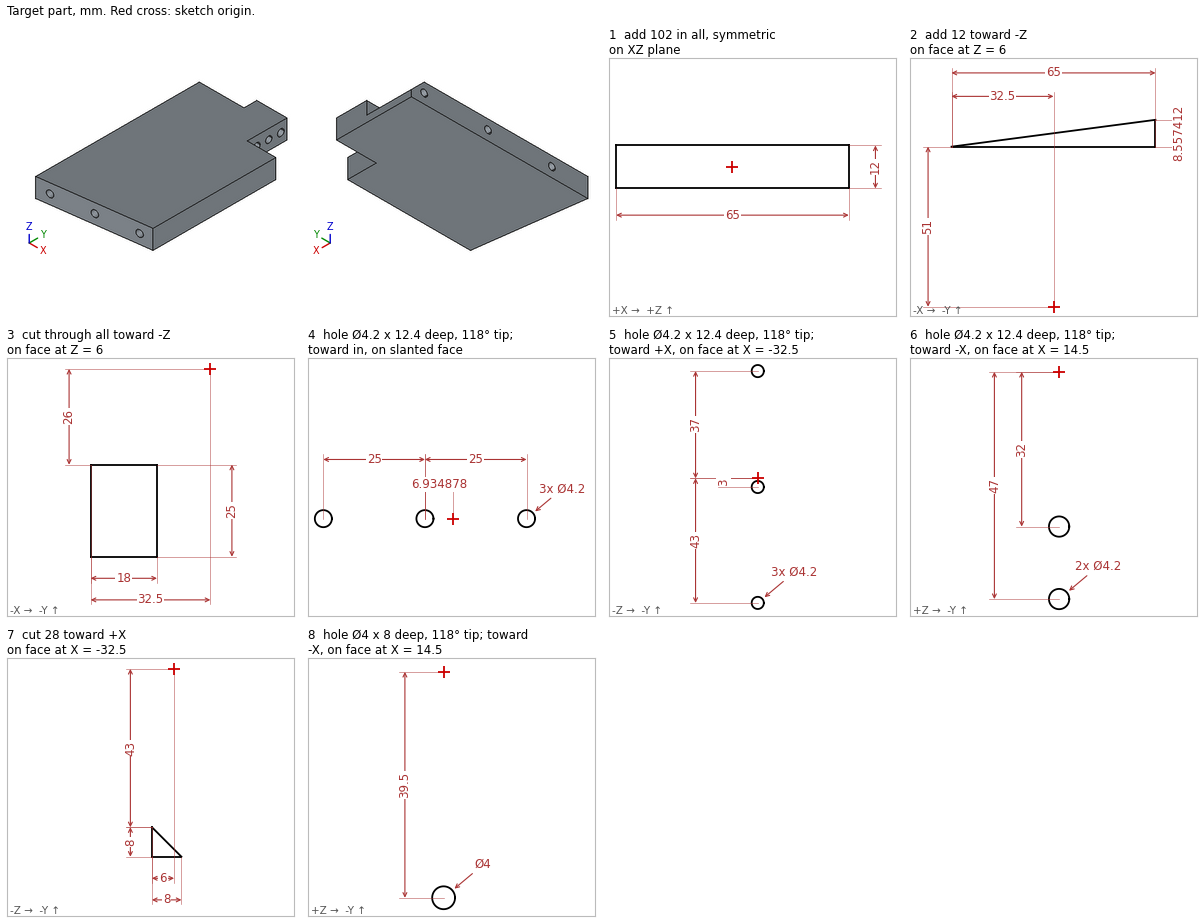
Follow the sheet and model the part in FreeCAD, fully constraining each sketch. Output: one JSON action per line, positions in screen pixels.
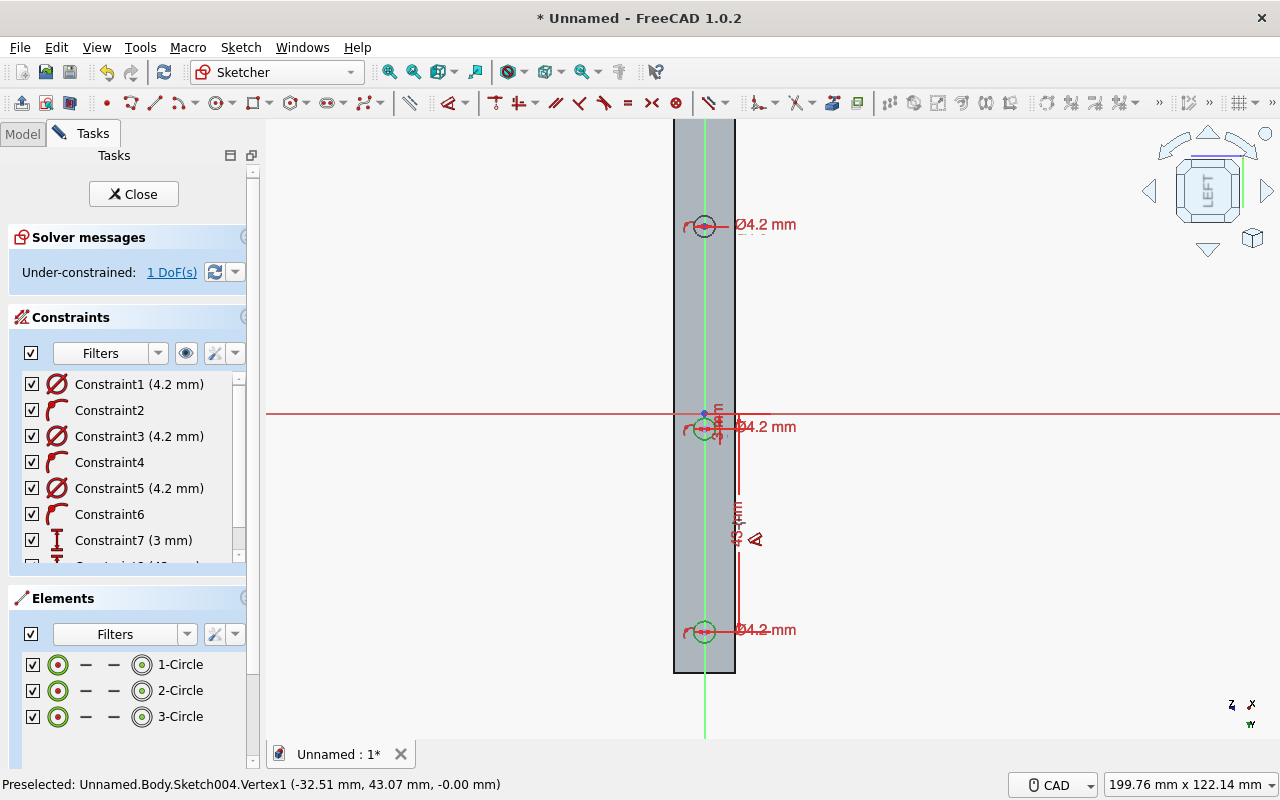
{"action": "left_click", "coordinate": [705, 227]}
{"action": "left_click", "coordinate": [739, 320]}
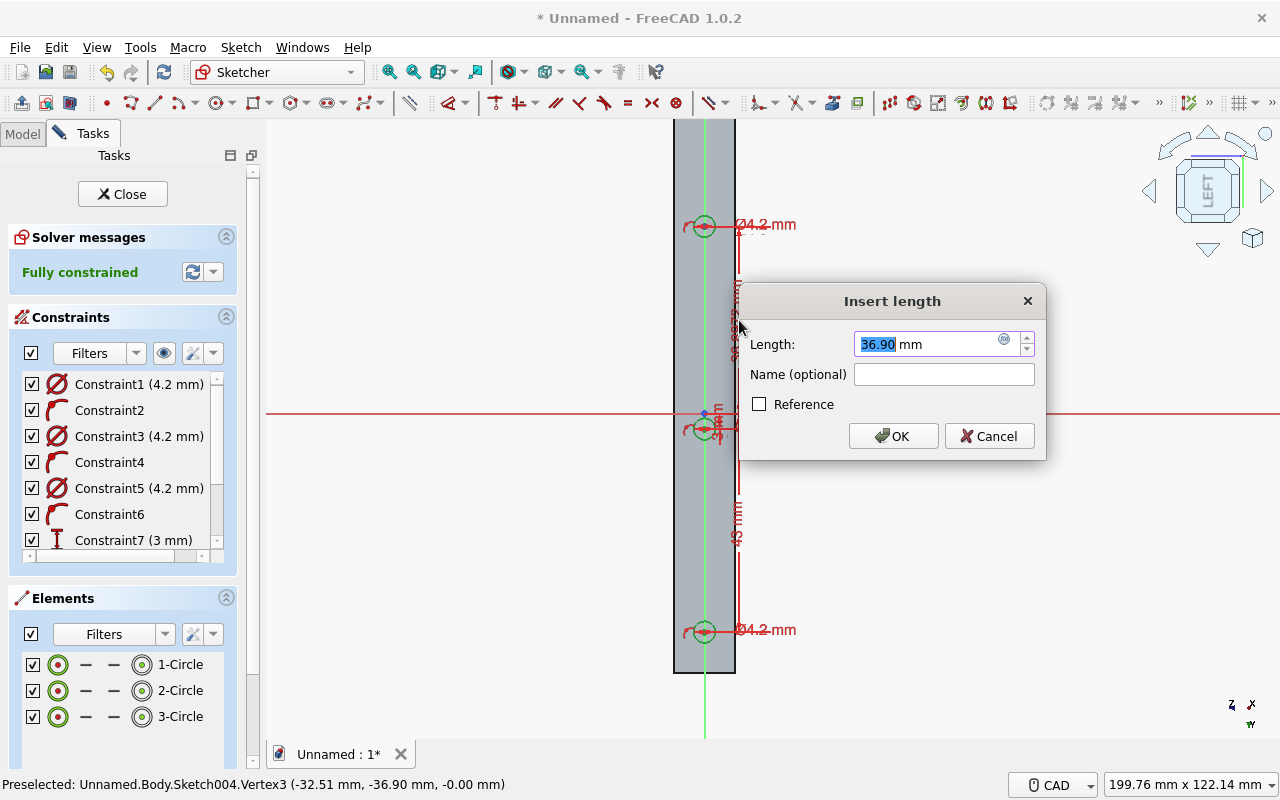
{"action": "type", "text": "37"}
{"action": "key", "text": "Return"}
{"action": "key", "text": "Escape"}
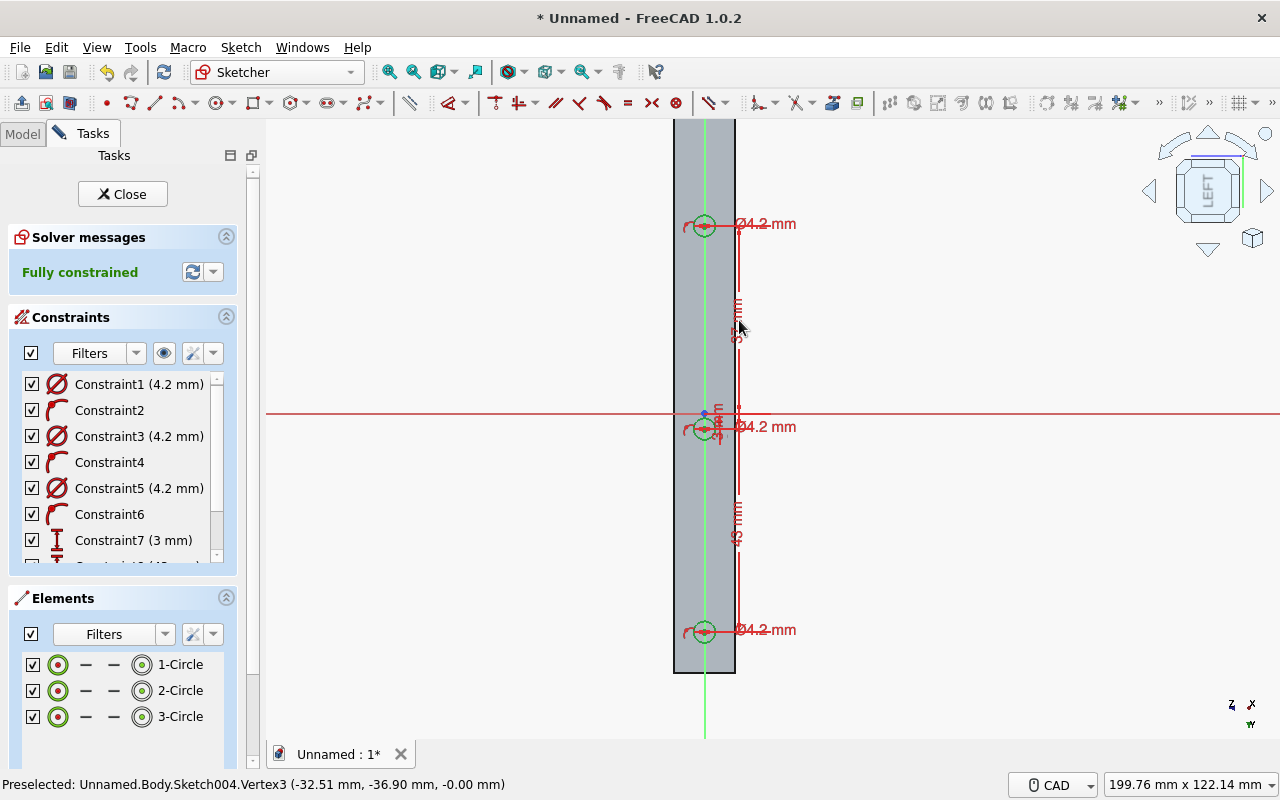
{"action": "left_click", "coordinate": [123, 194]}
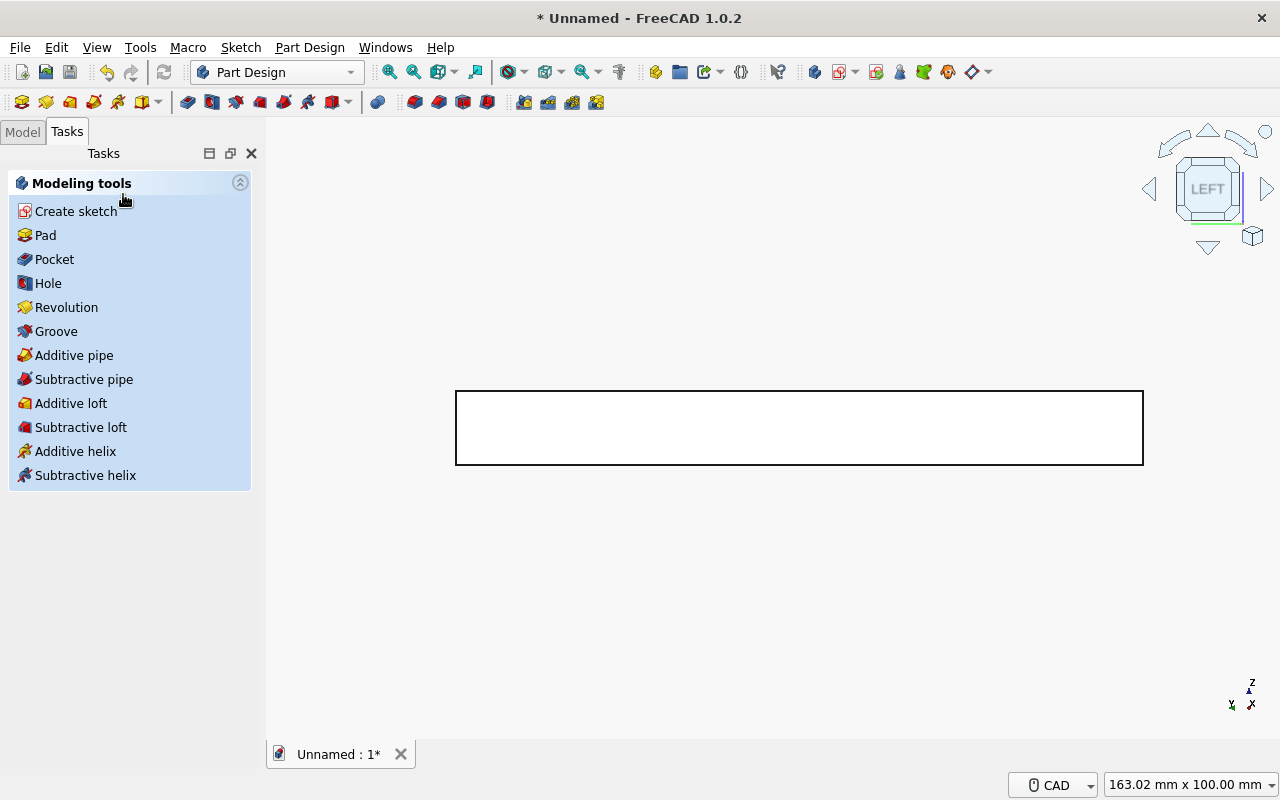
{"action": "left_click", "coordinate": [212, 102]}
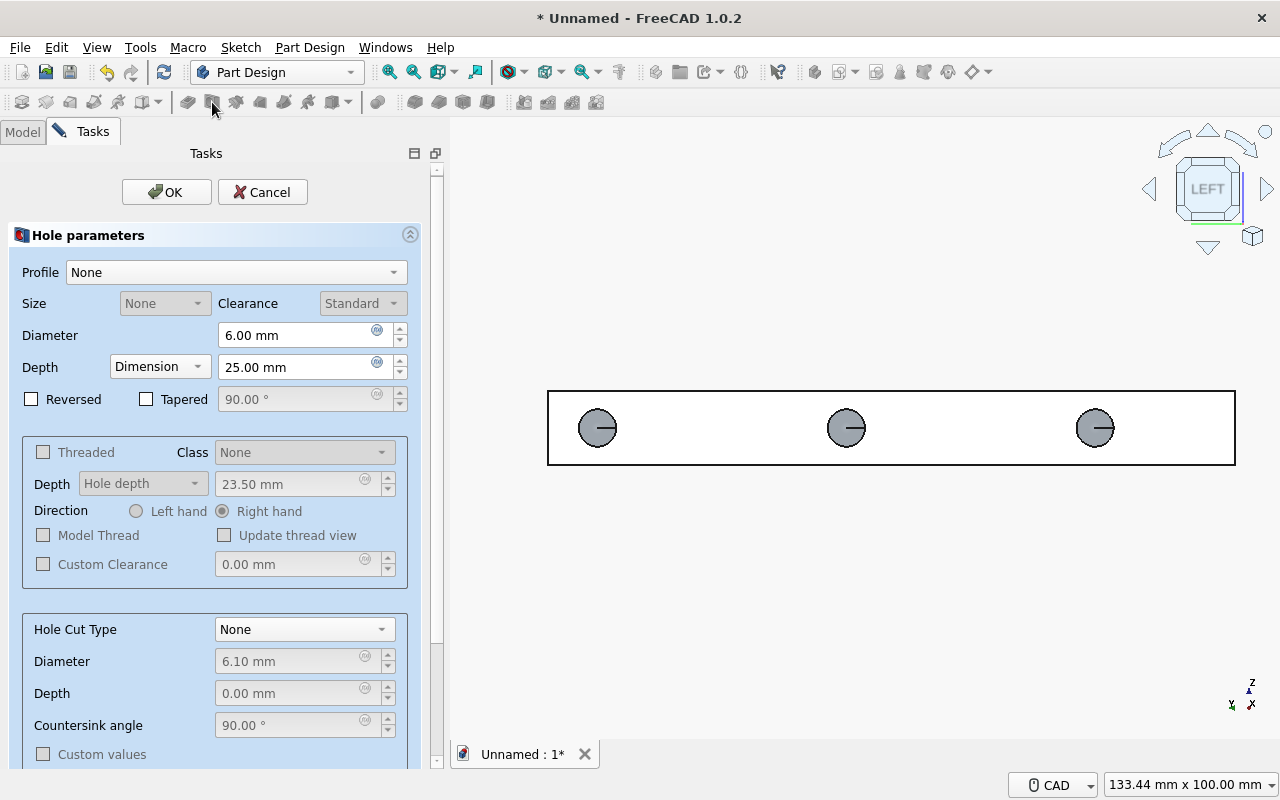
{"action": "triple_click", "coordinate": [305, 335]}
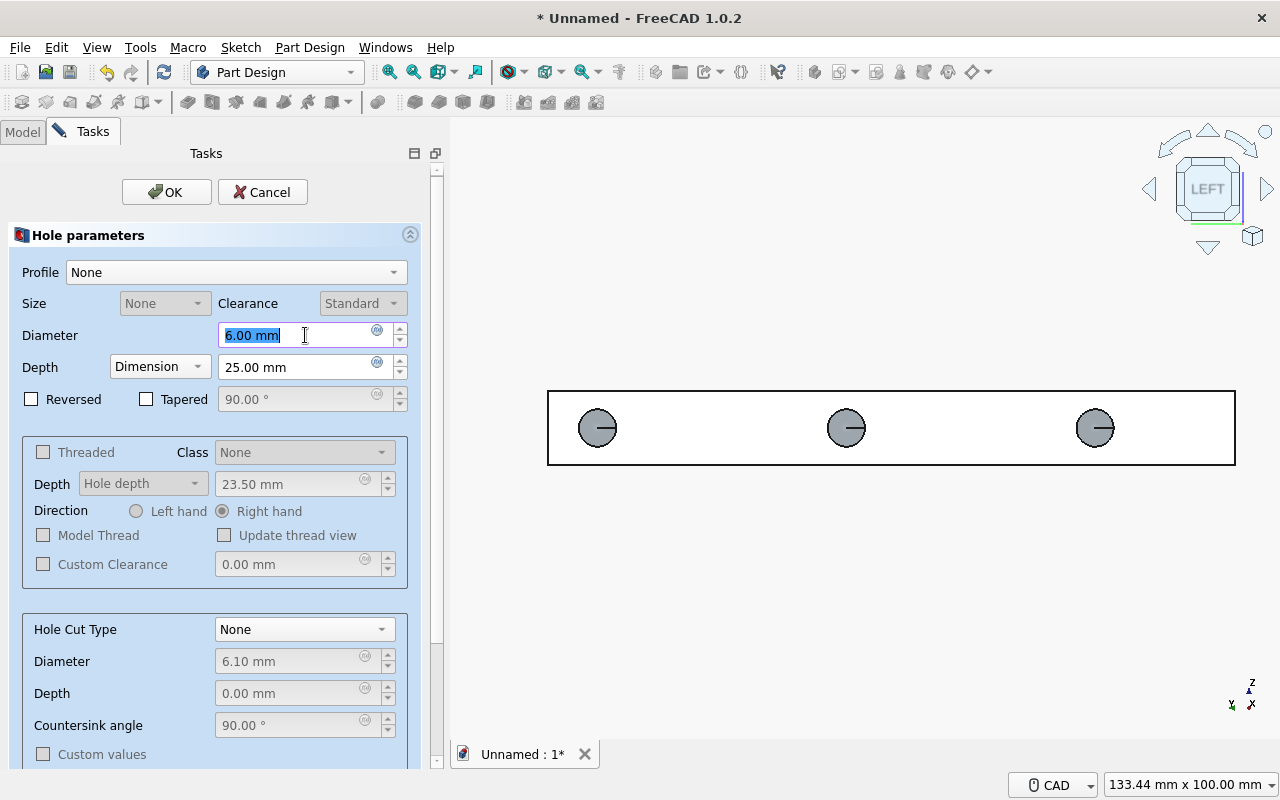
{"action": "type", "text": "4.2"}
{"action": "key", "text": "Tab"}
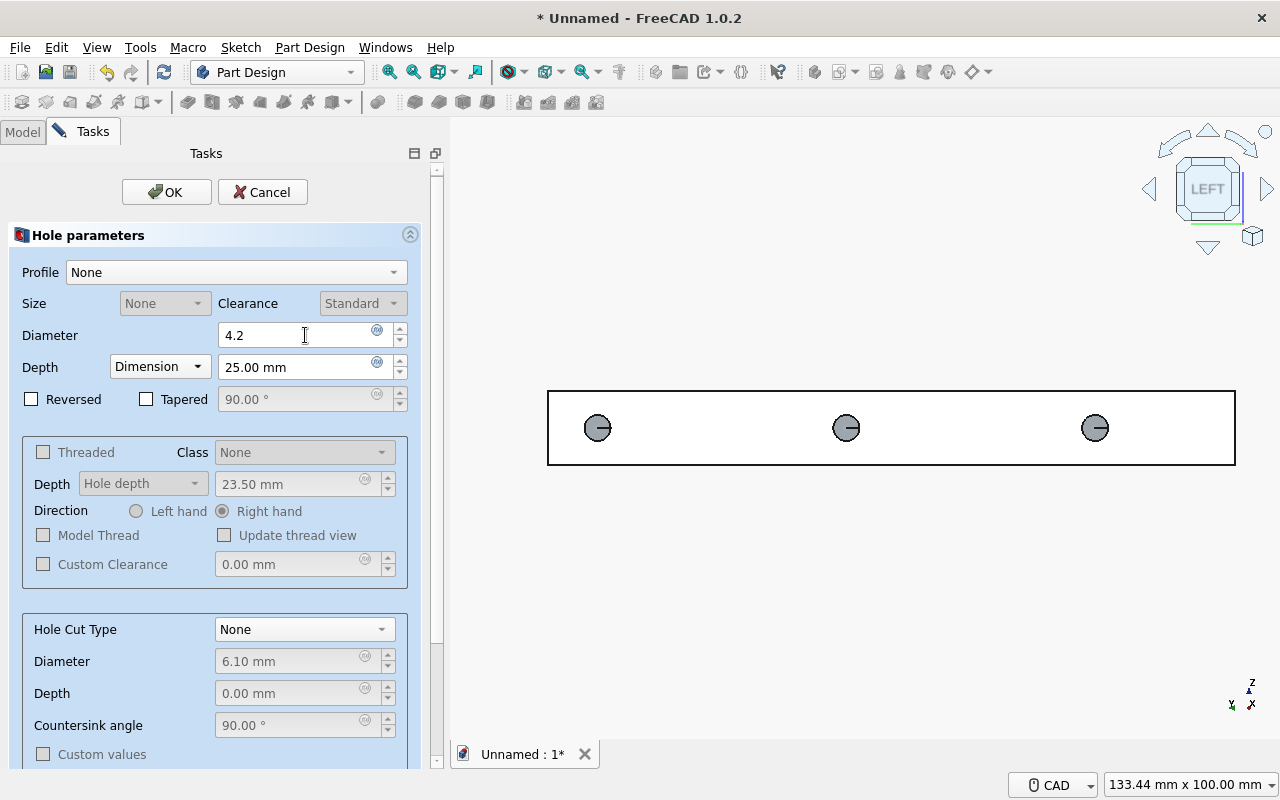
{"action": "triple_click", "coordinate": [305, 367]}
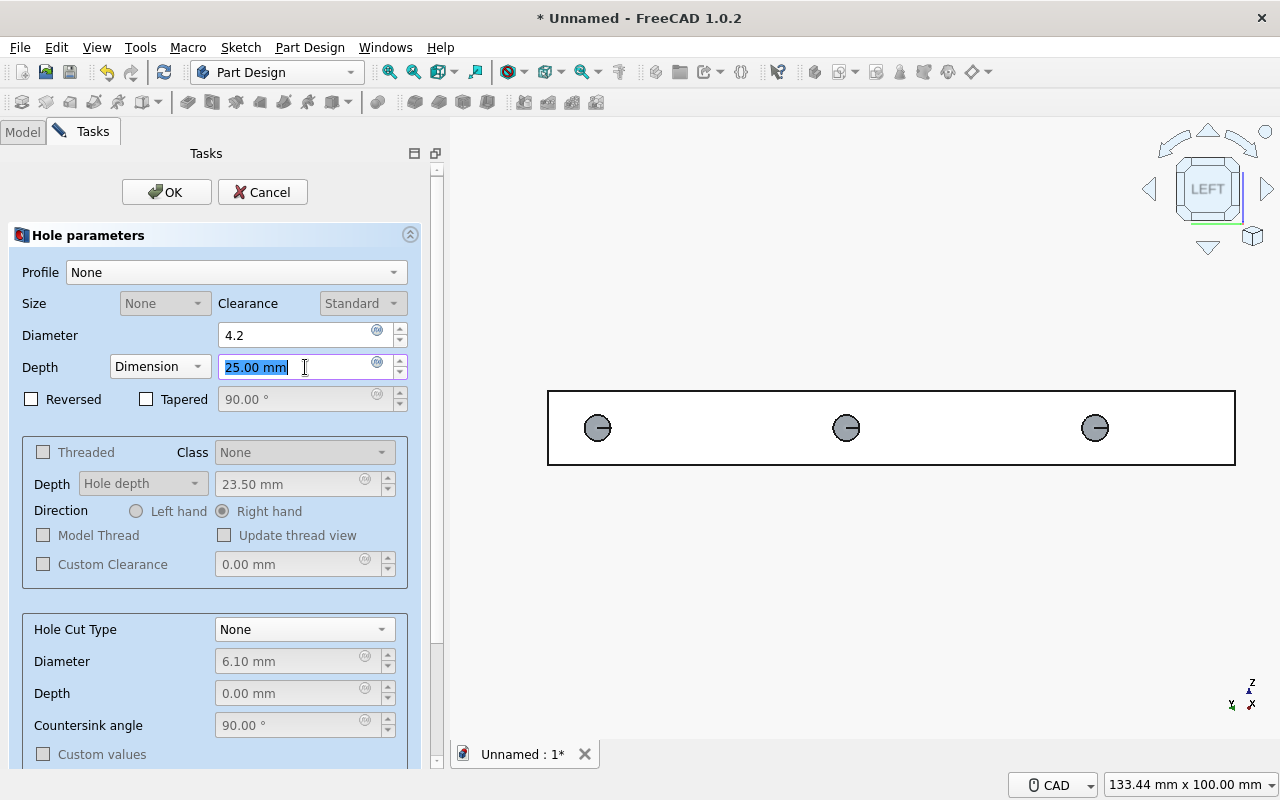
{"action": "type", "text": "12.4"}
{"action": "key", "text": "Tab"}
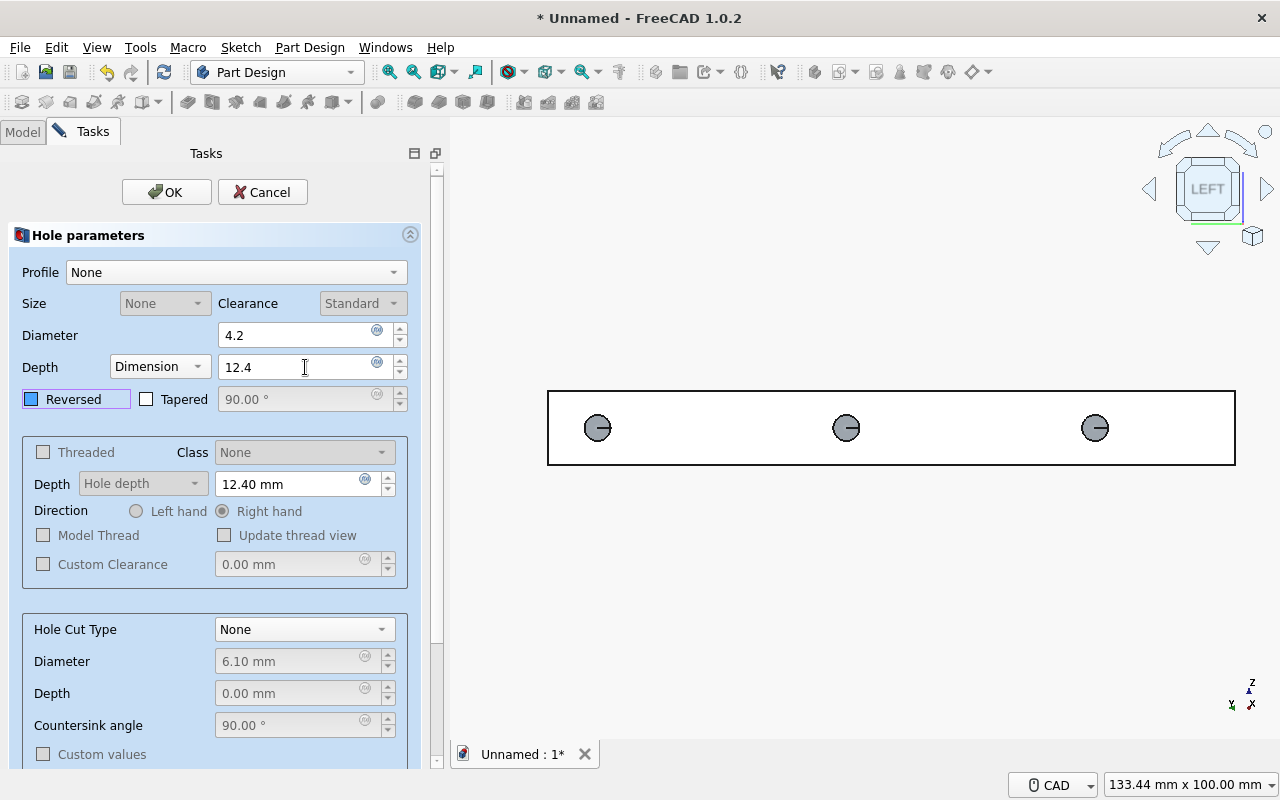
{"action": "left_click", "coordinate": [167, 192]}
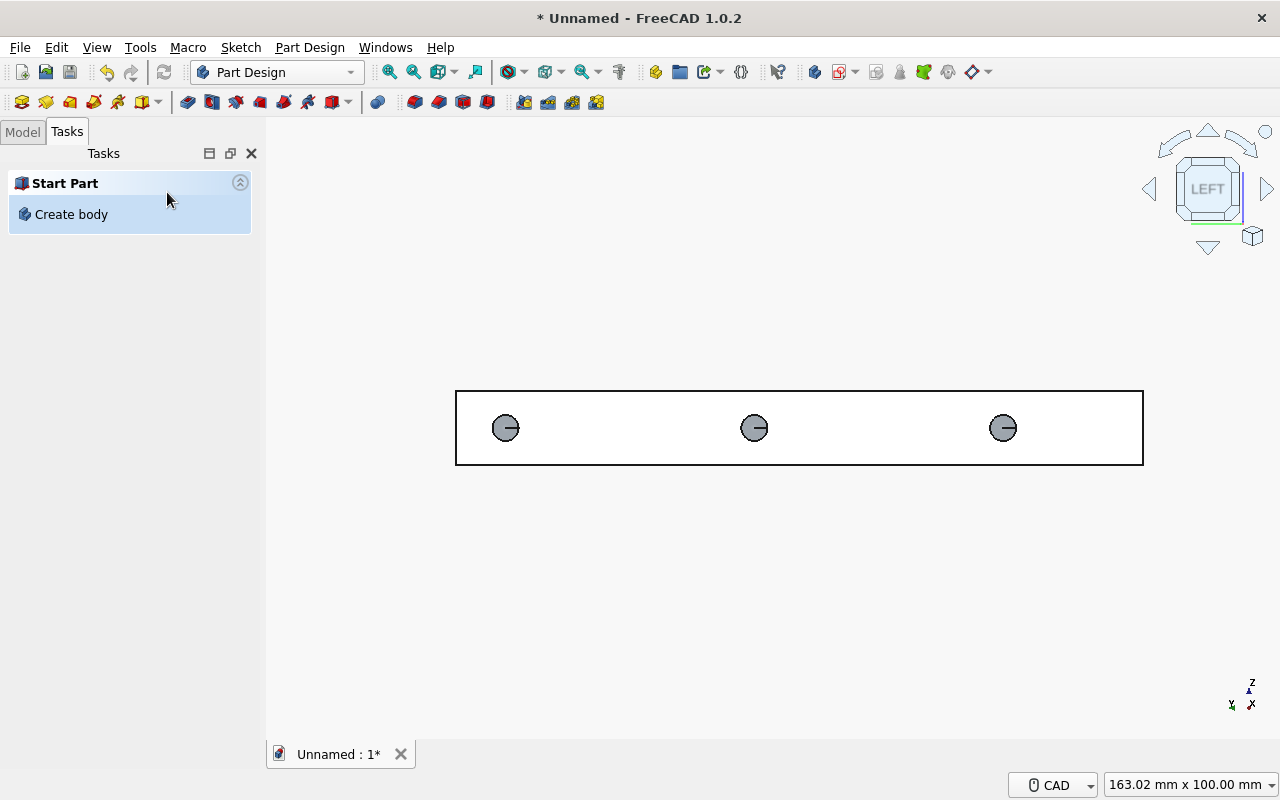
{"action": "key", "text": "0"}